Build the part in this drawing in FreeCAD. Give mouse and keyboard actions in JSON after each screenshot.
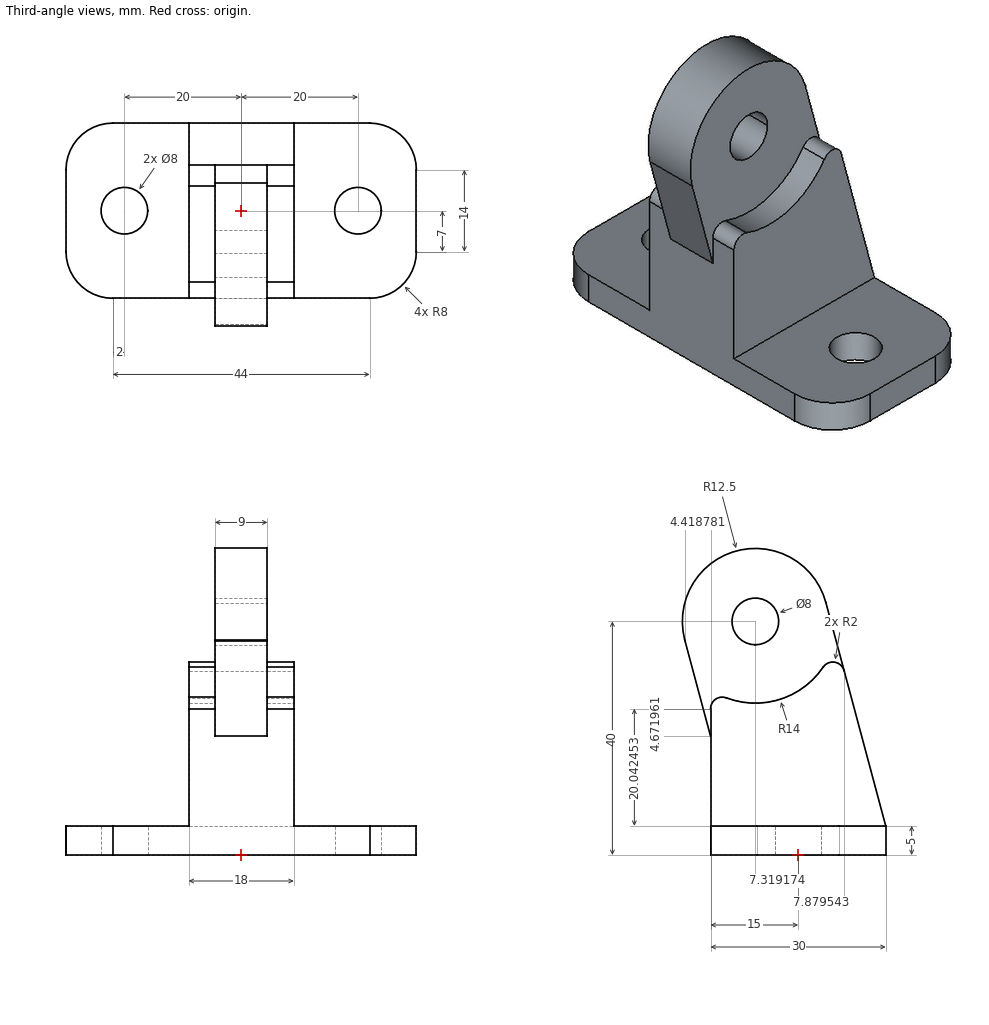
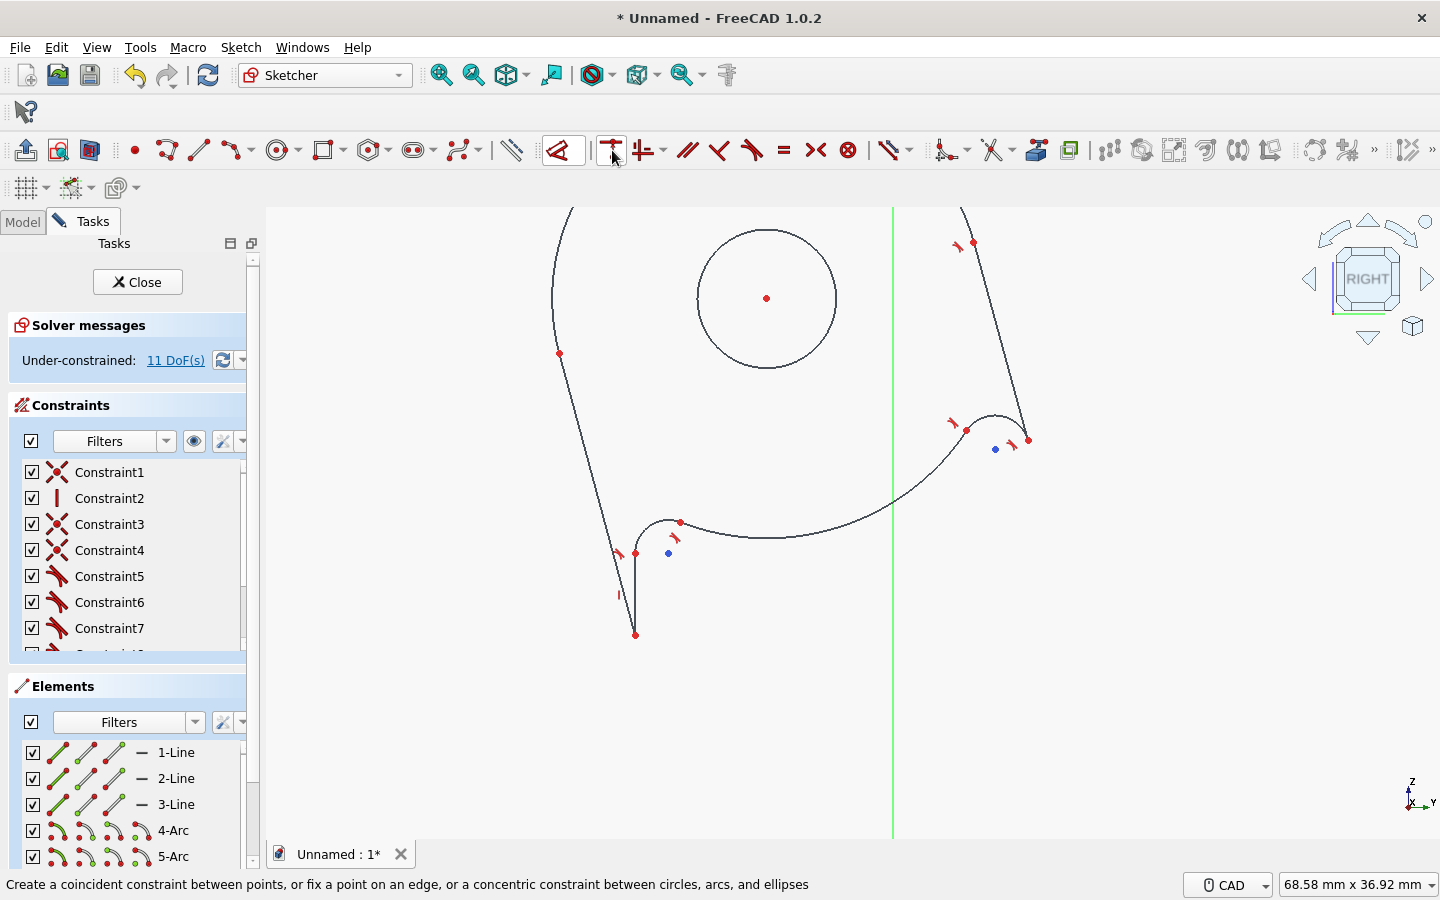
{"action": "left_click", "coordinate": [662, 521]}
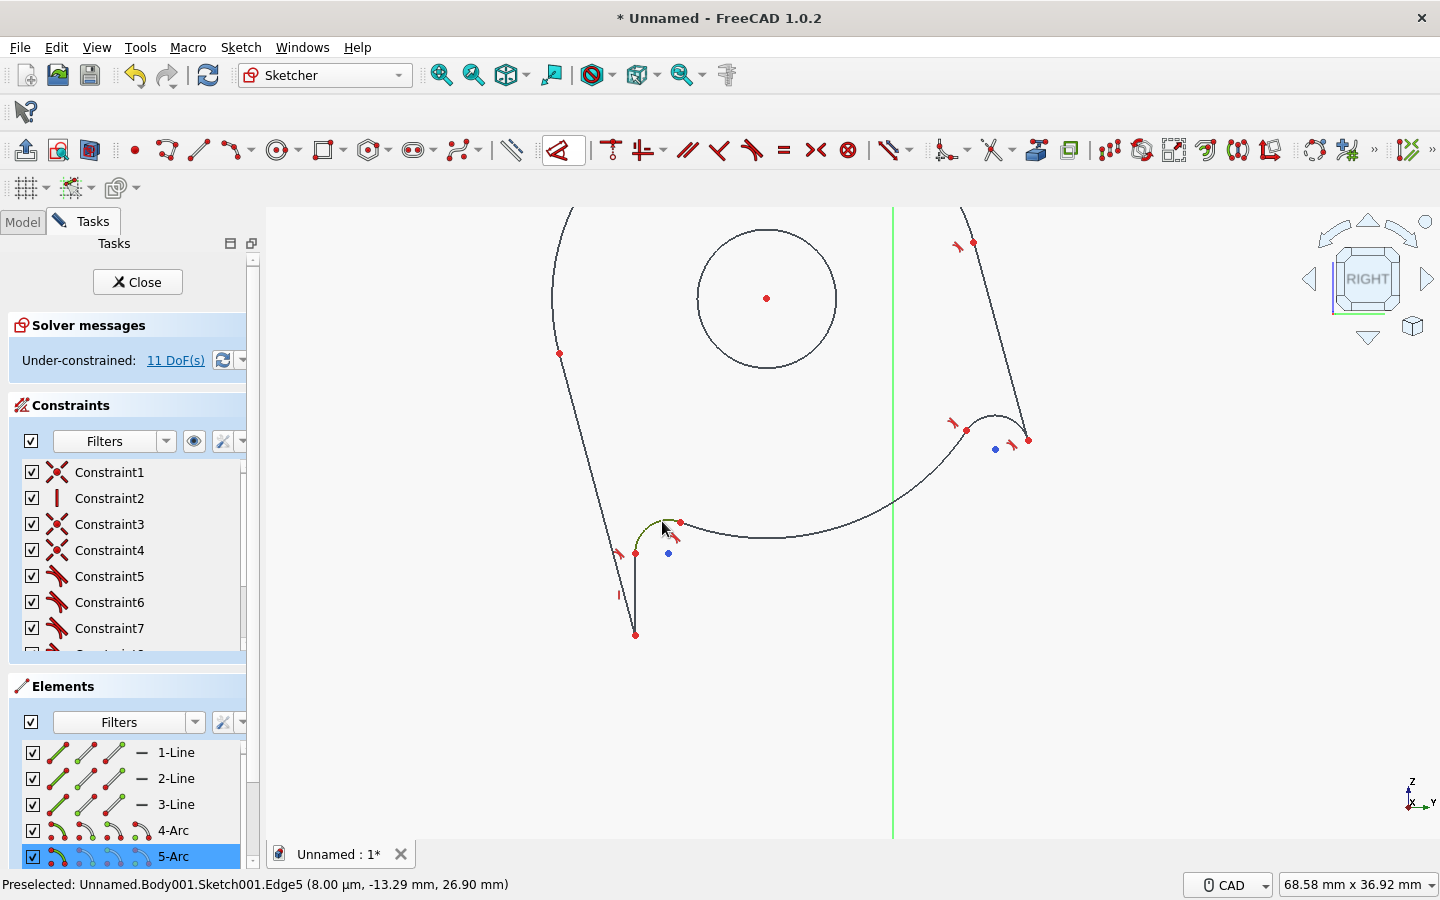
{"action": "left_click", "coordinate": [985, 417]}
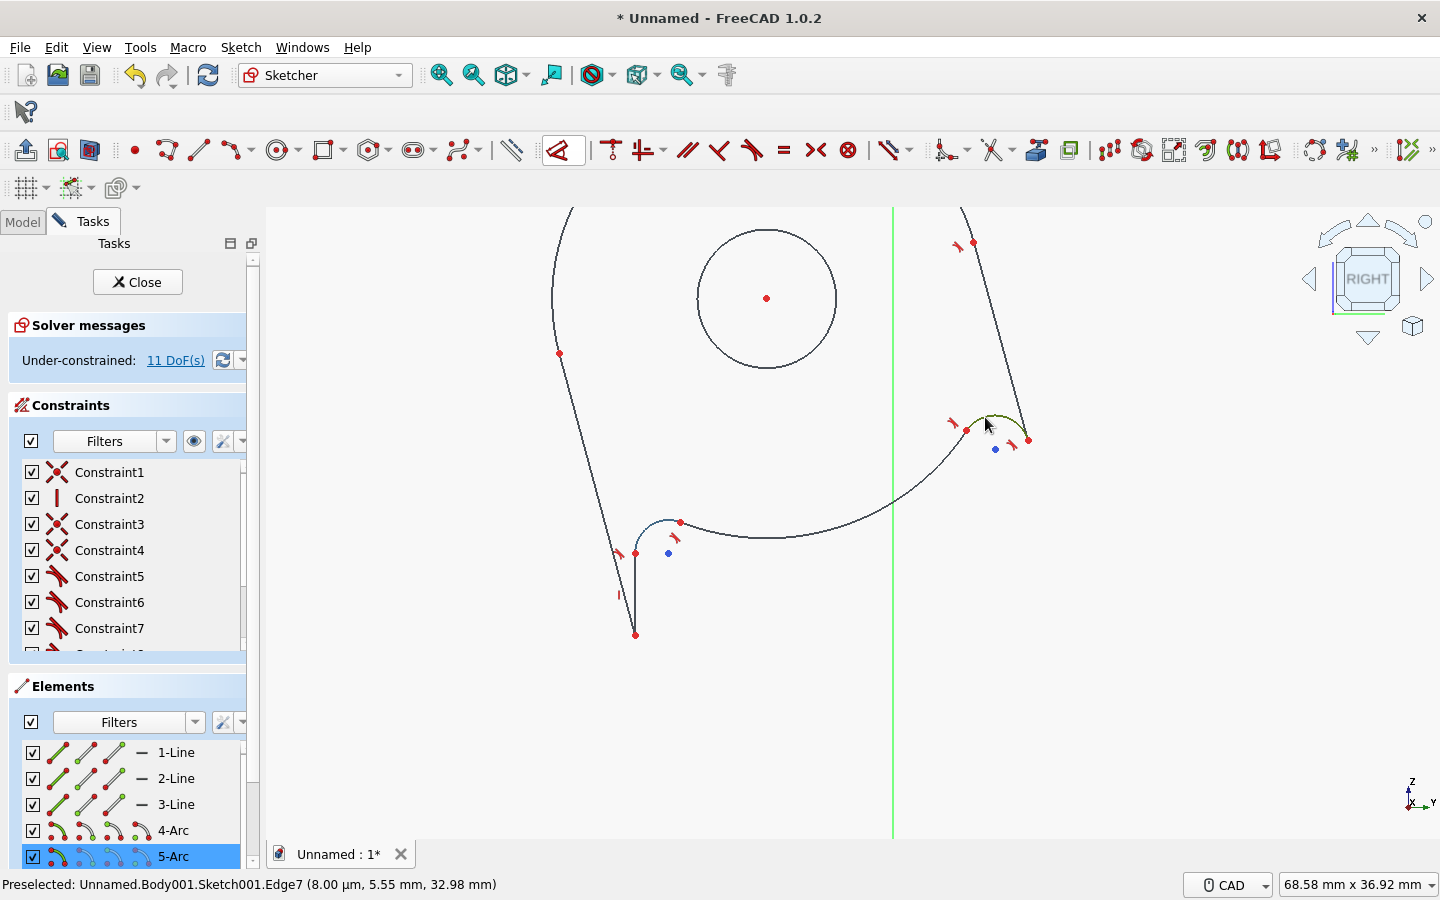
{"action": "key", "text": "e"}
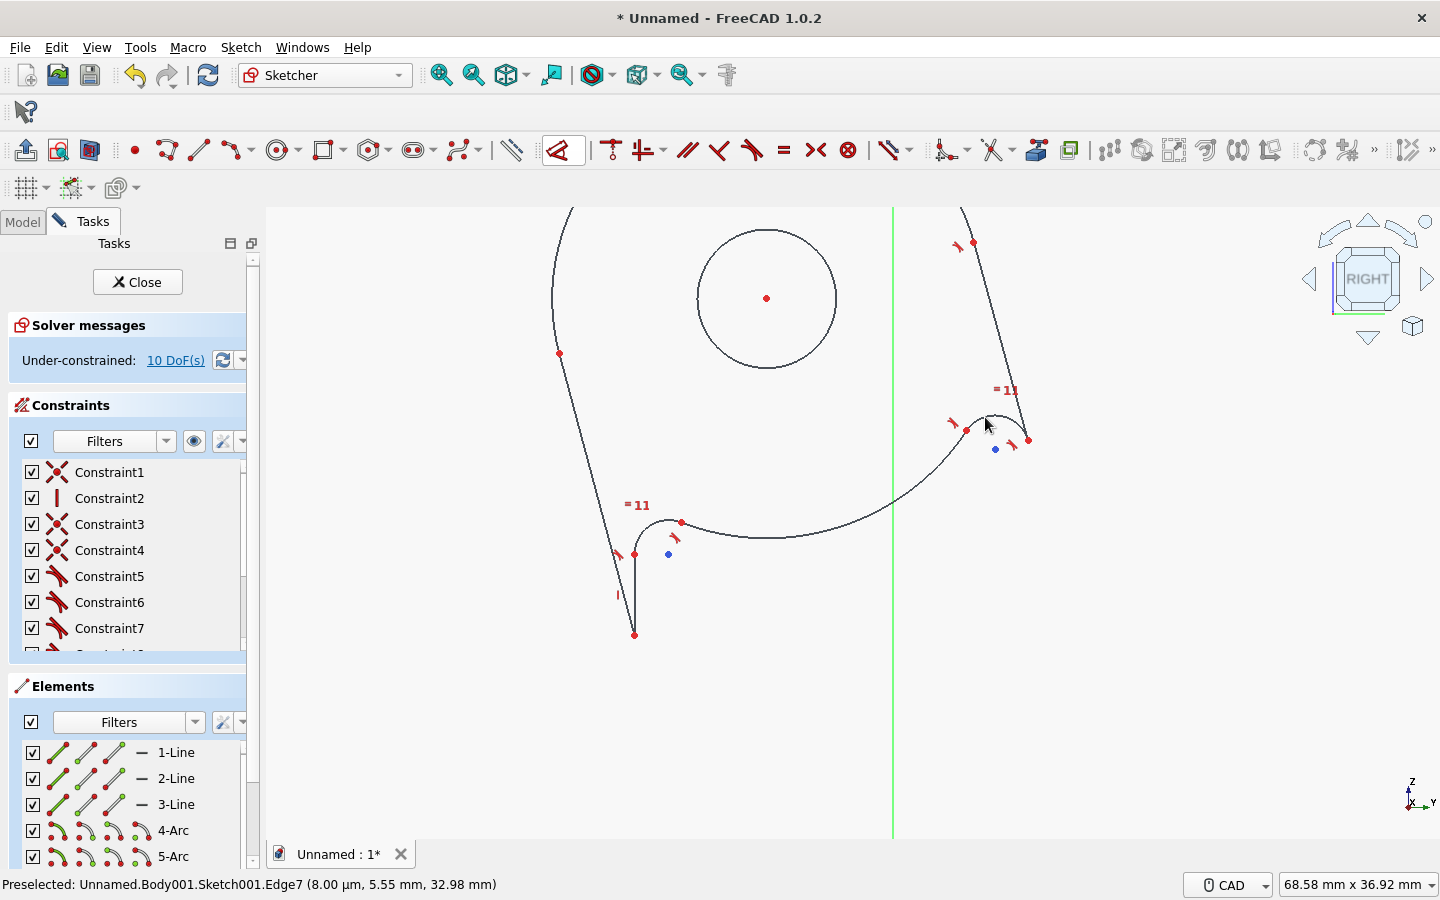
{"action": "scroll", "coordinate": [777, 513], "scroll_direction": "down", "scroll_amount": 4}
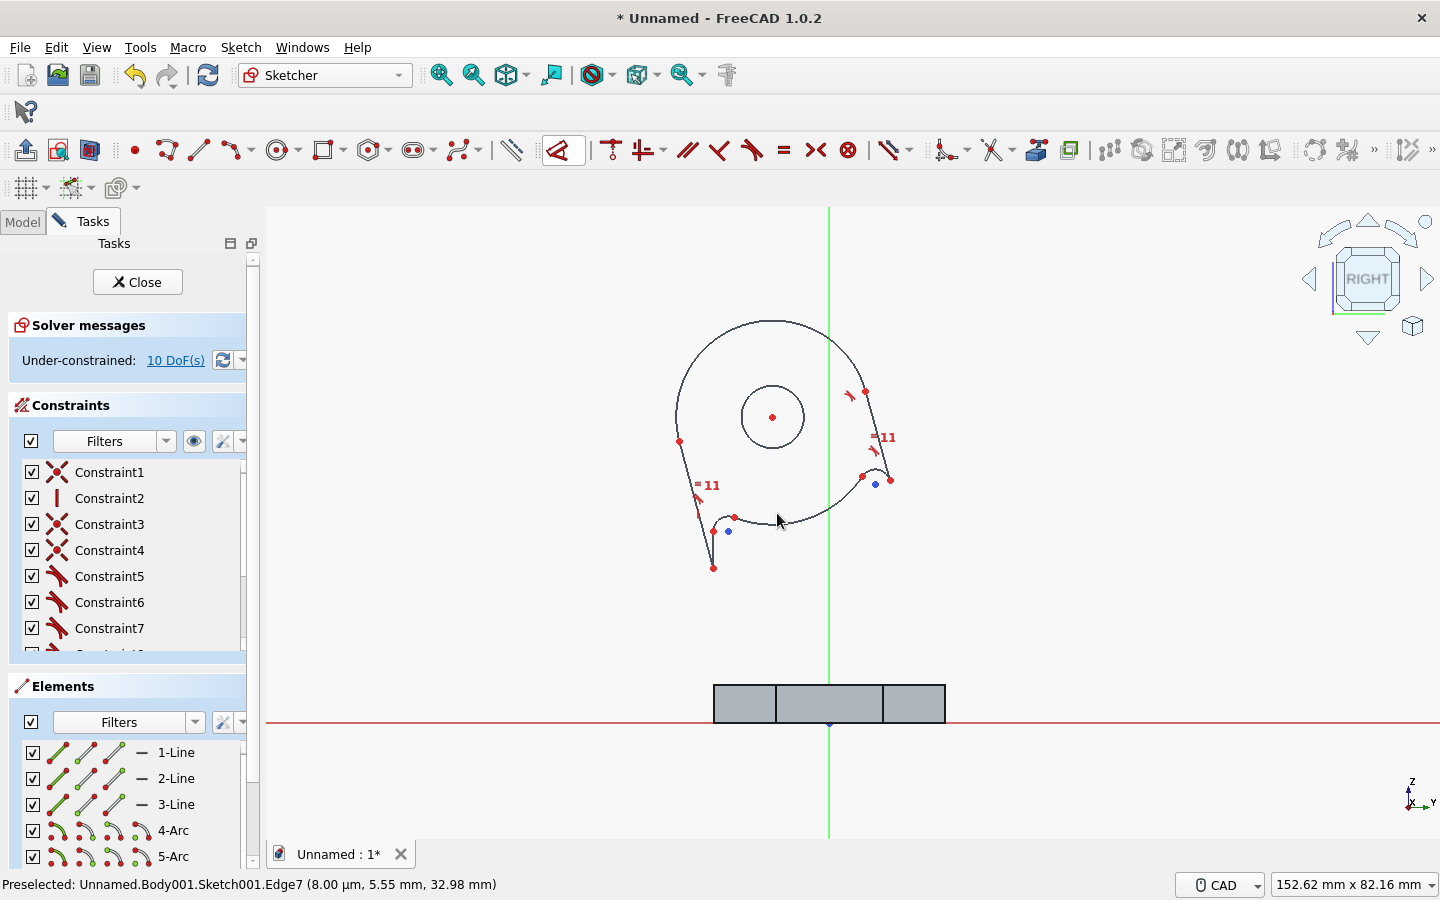
{"action": "left_click", "coordinate": [807, 327]}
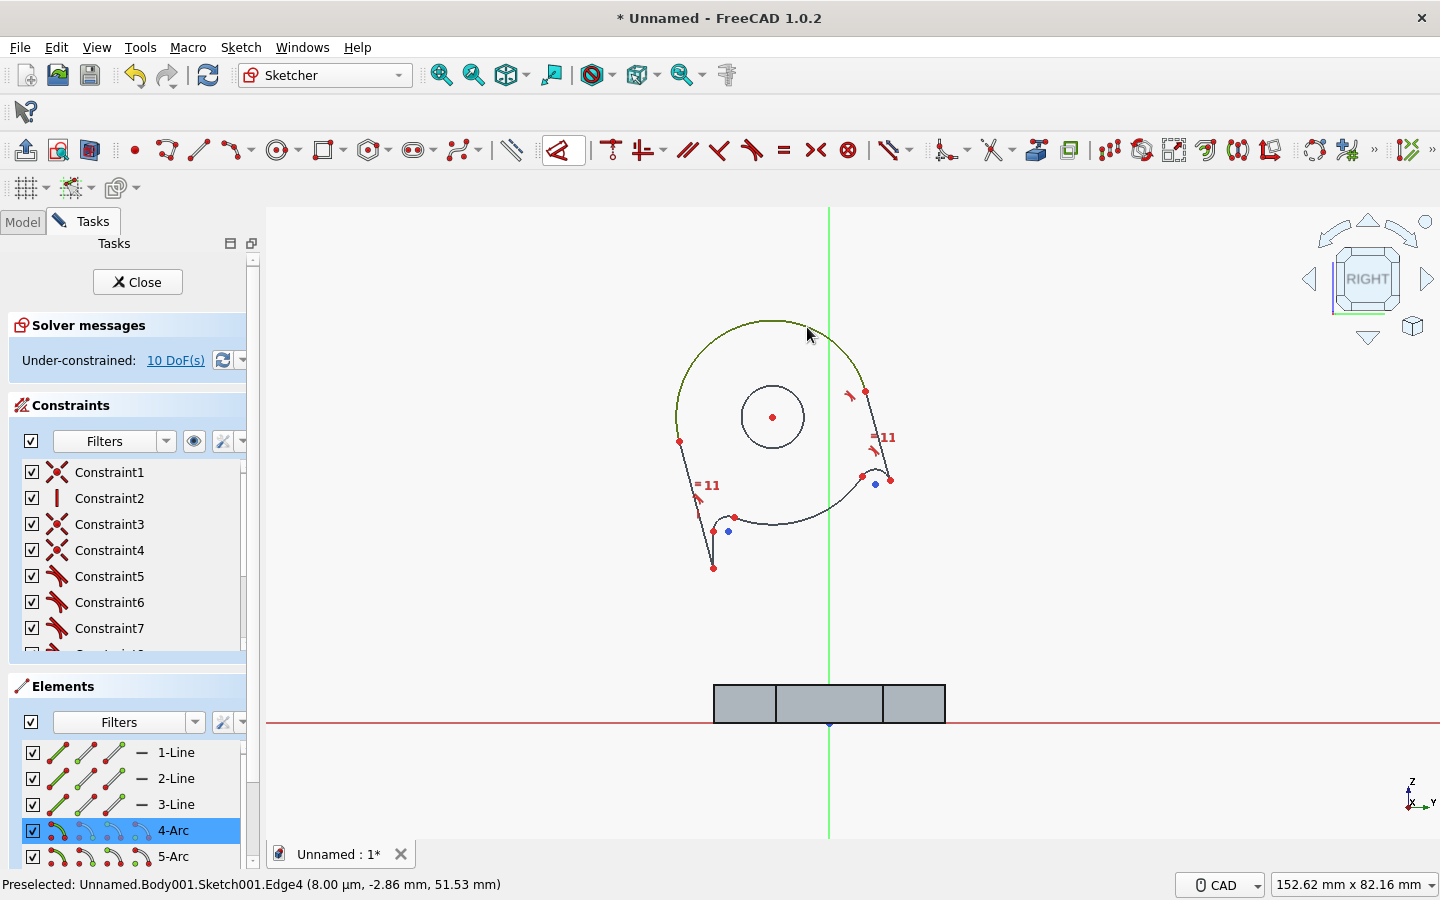
{"action": "key", "text": "k r"}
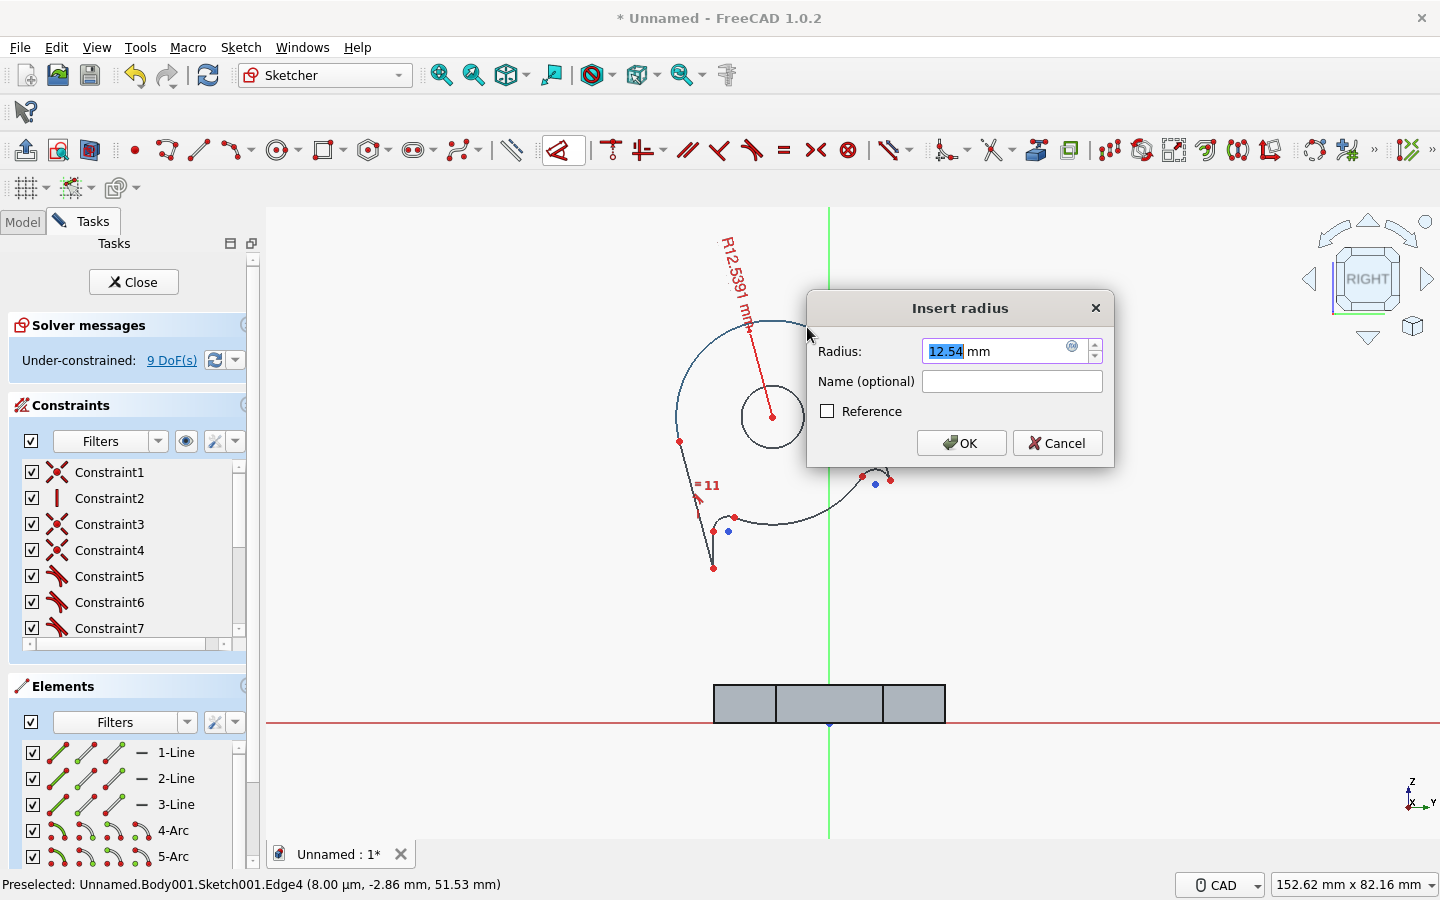
{"action": "type", "text": "12.5"}
{"action": "key", "text": "Return"}